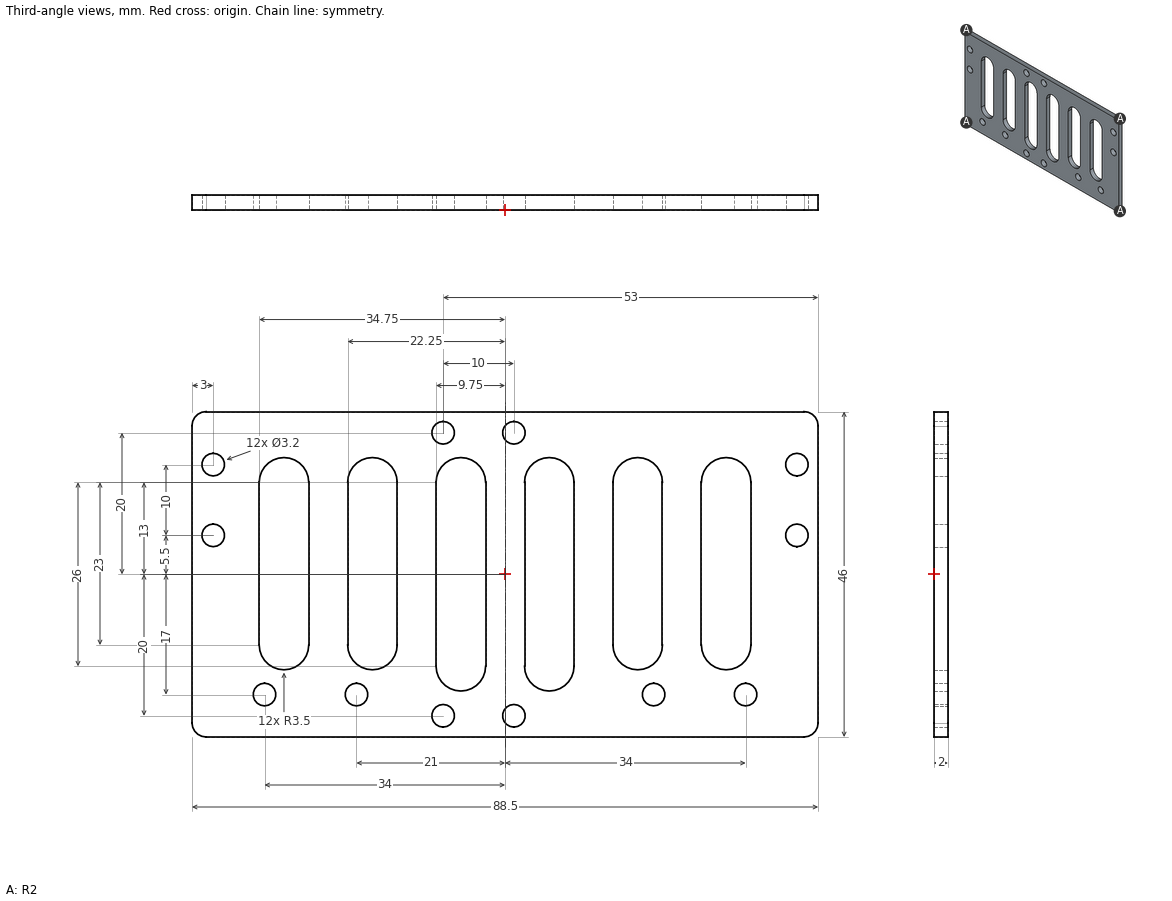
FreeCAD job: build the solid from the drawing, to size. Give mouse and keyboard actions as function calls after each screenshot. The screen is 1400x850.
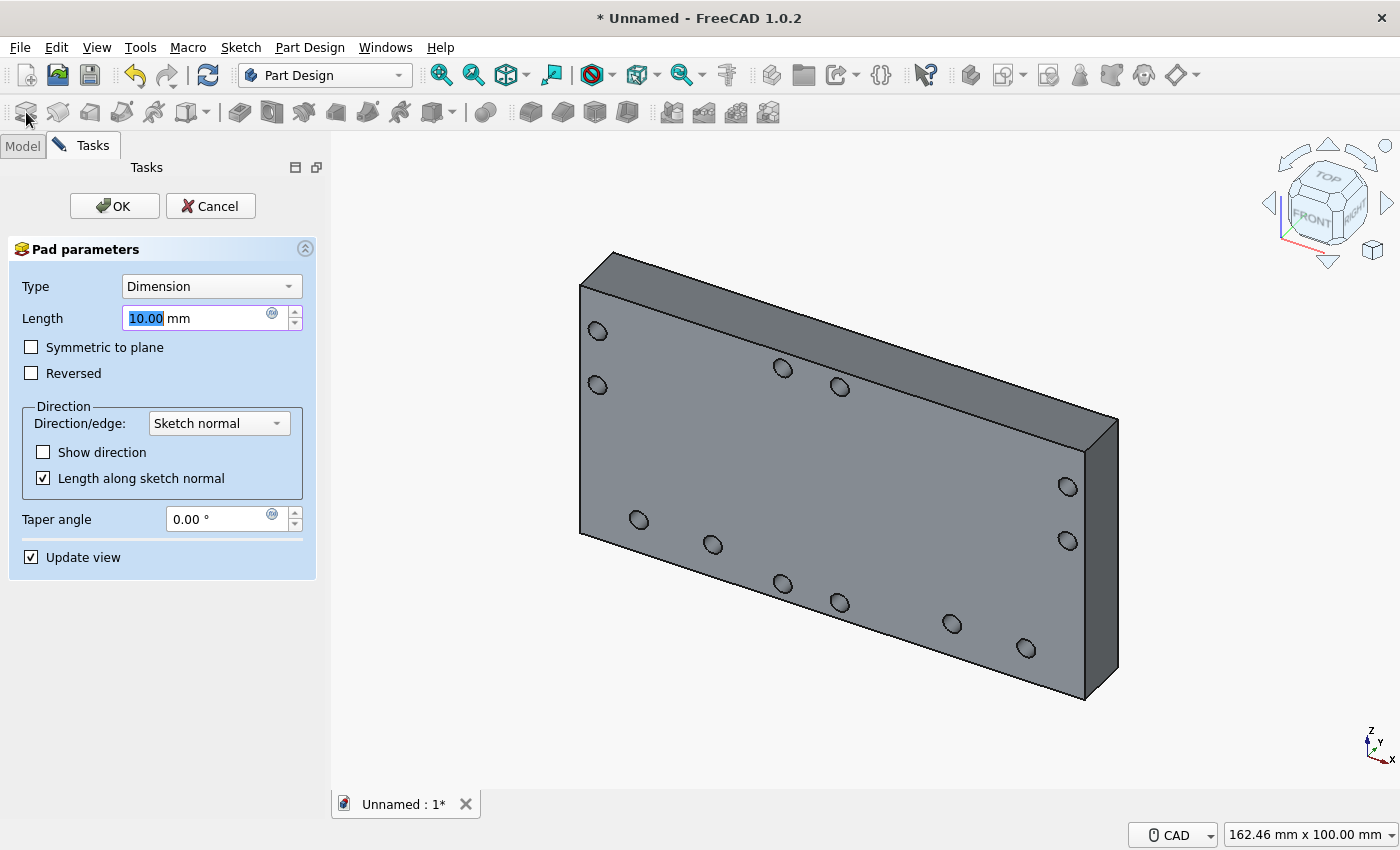
text(2)
key(Tab)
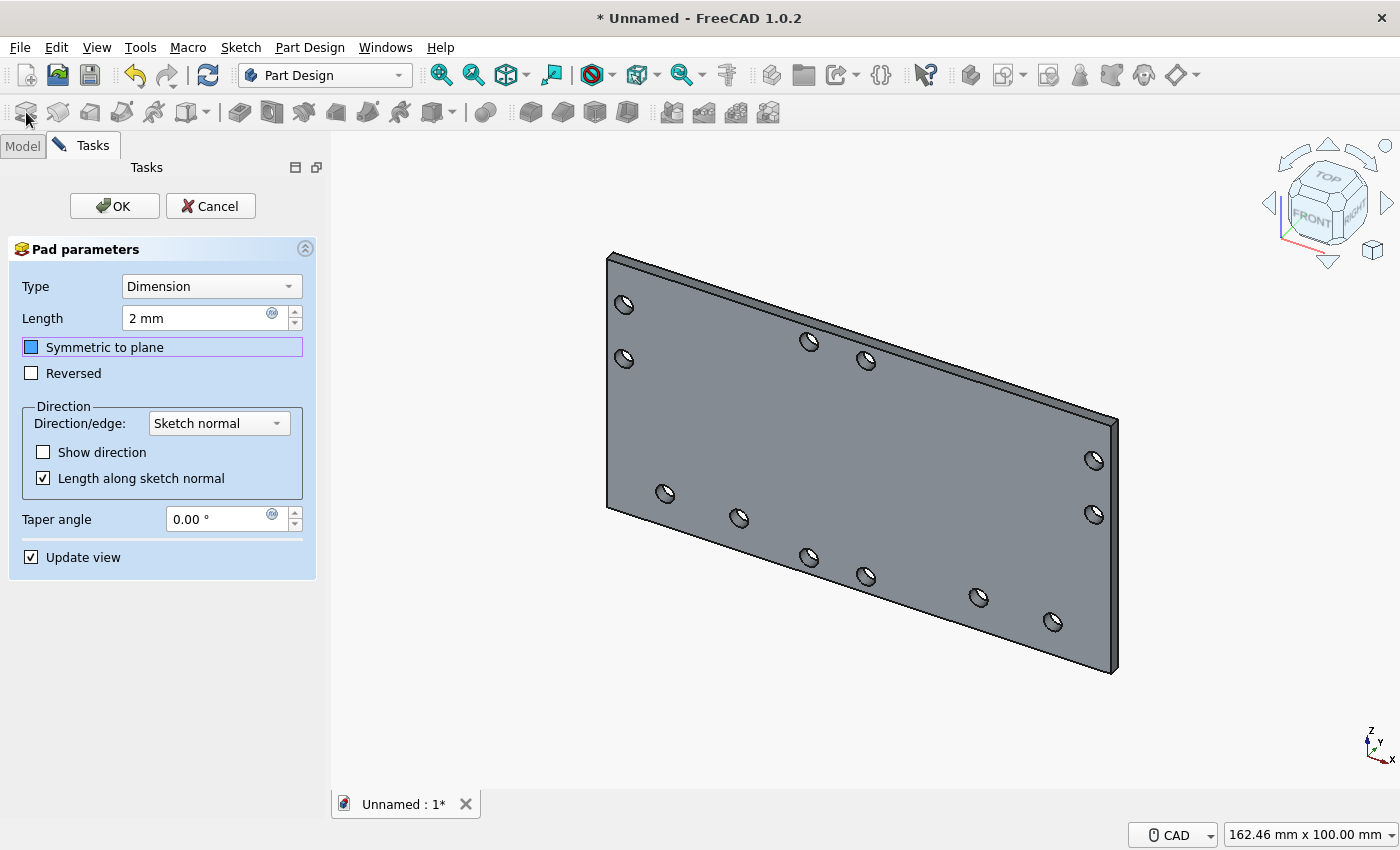
click(30, 373)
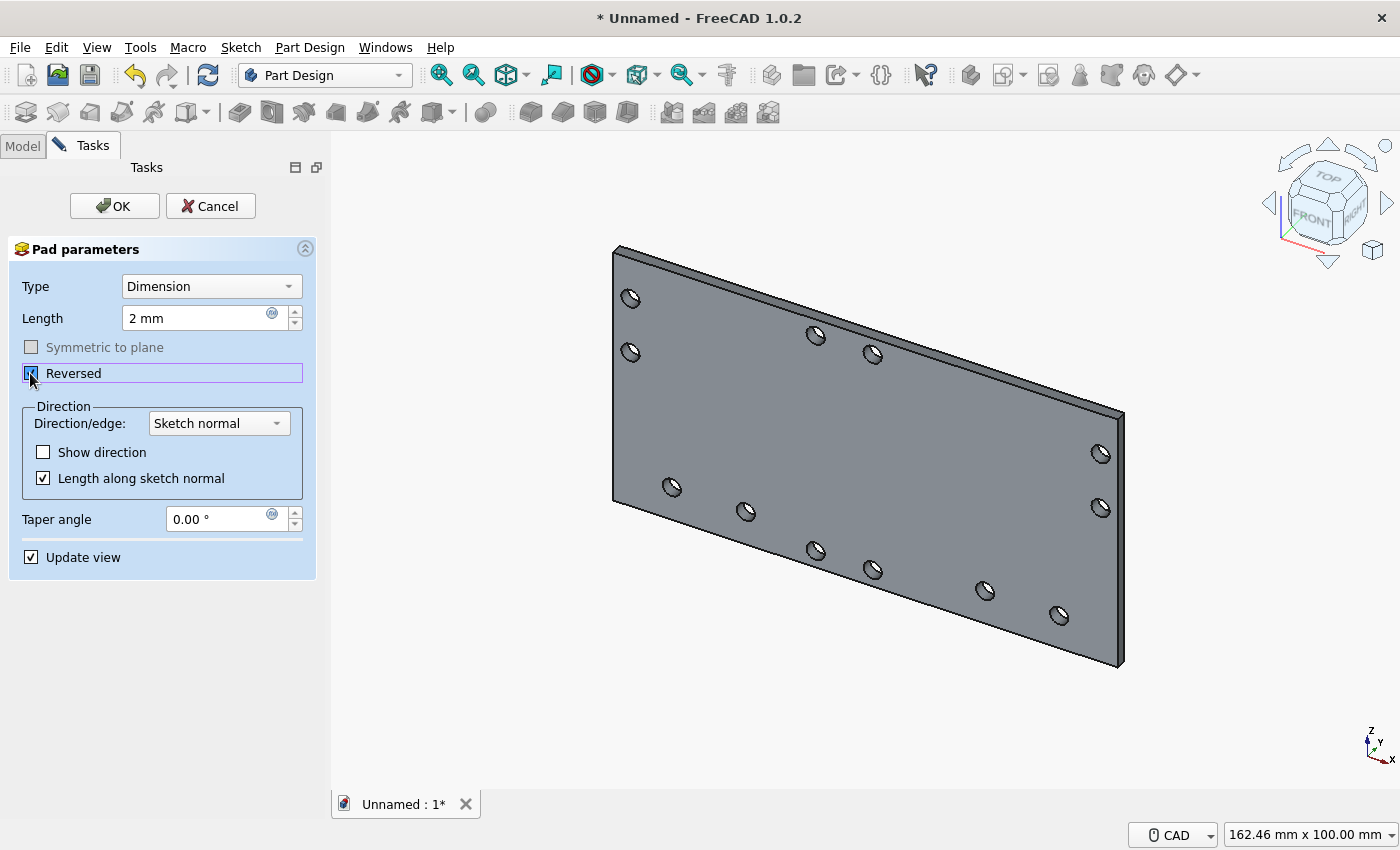
click(115, 206)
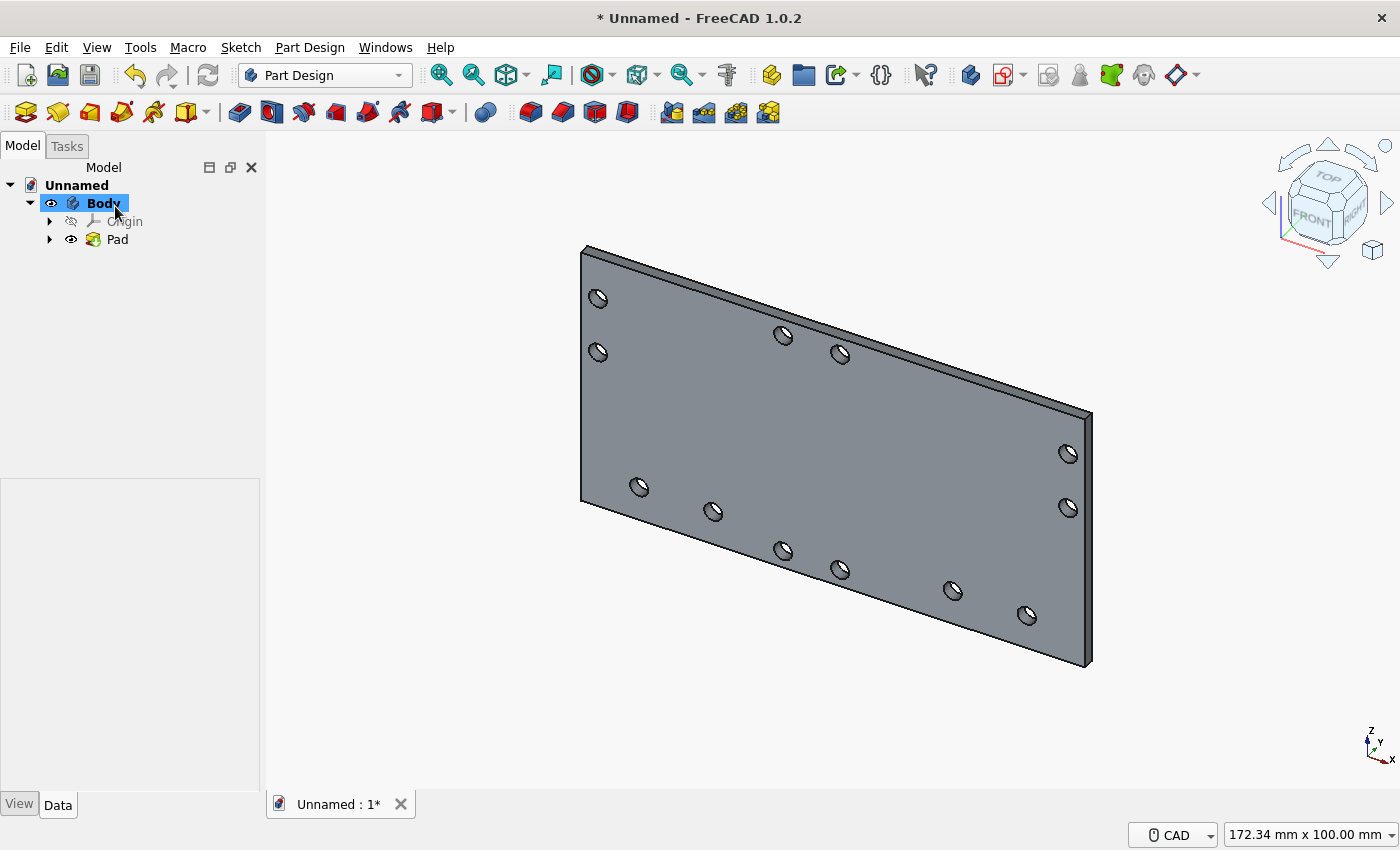
key(4)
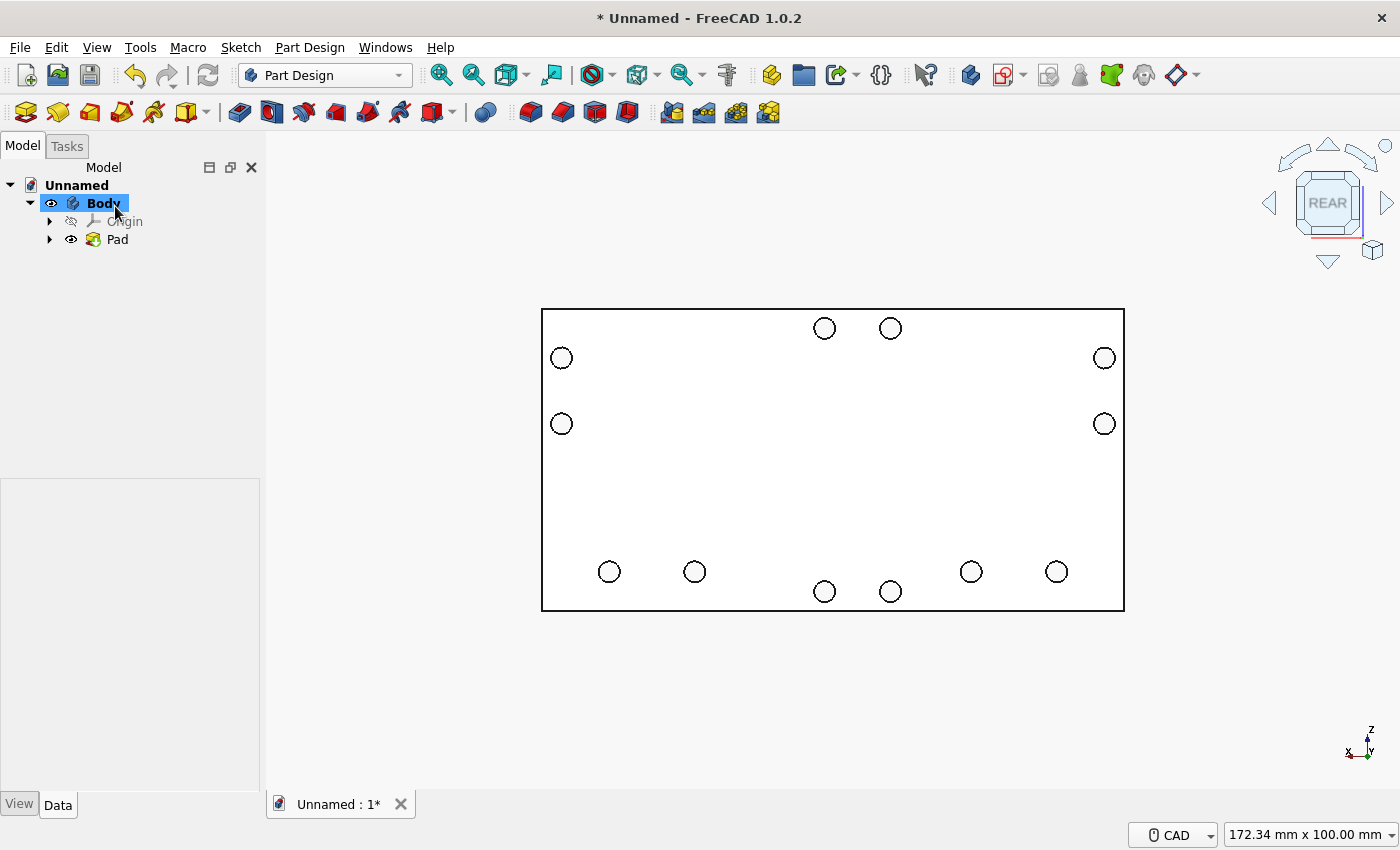
click(833, 459)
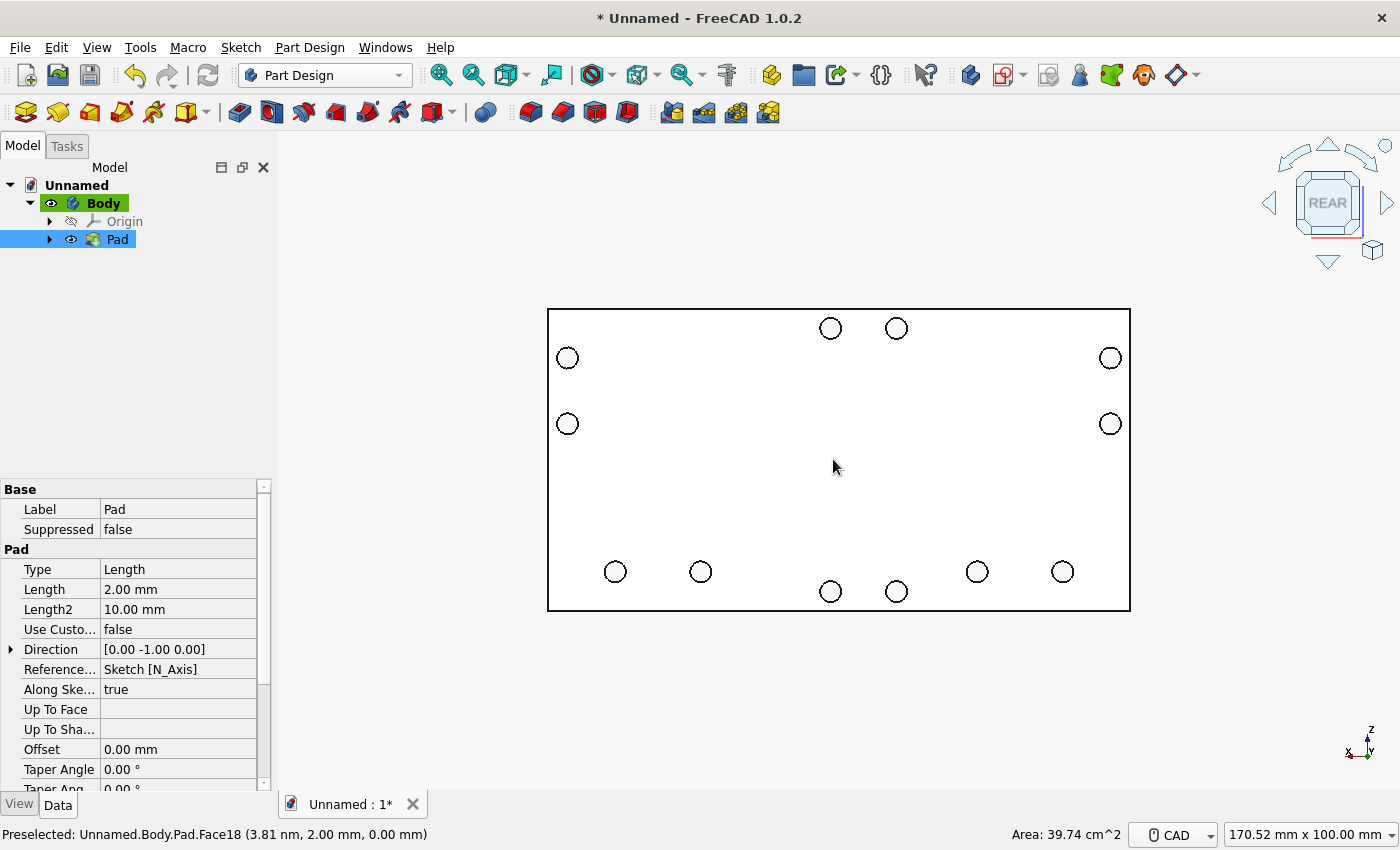
click(1004, 76)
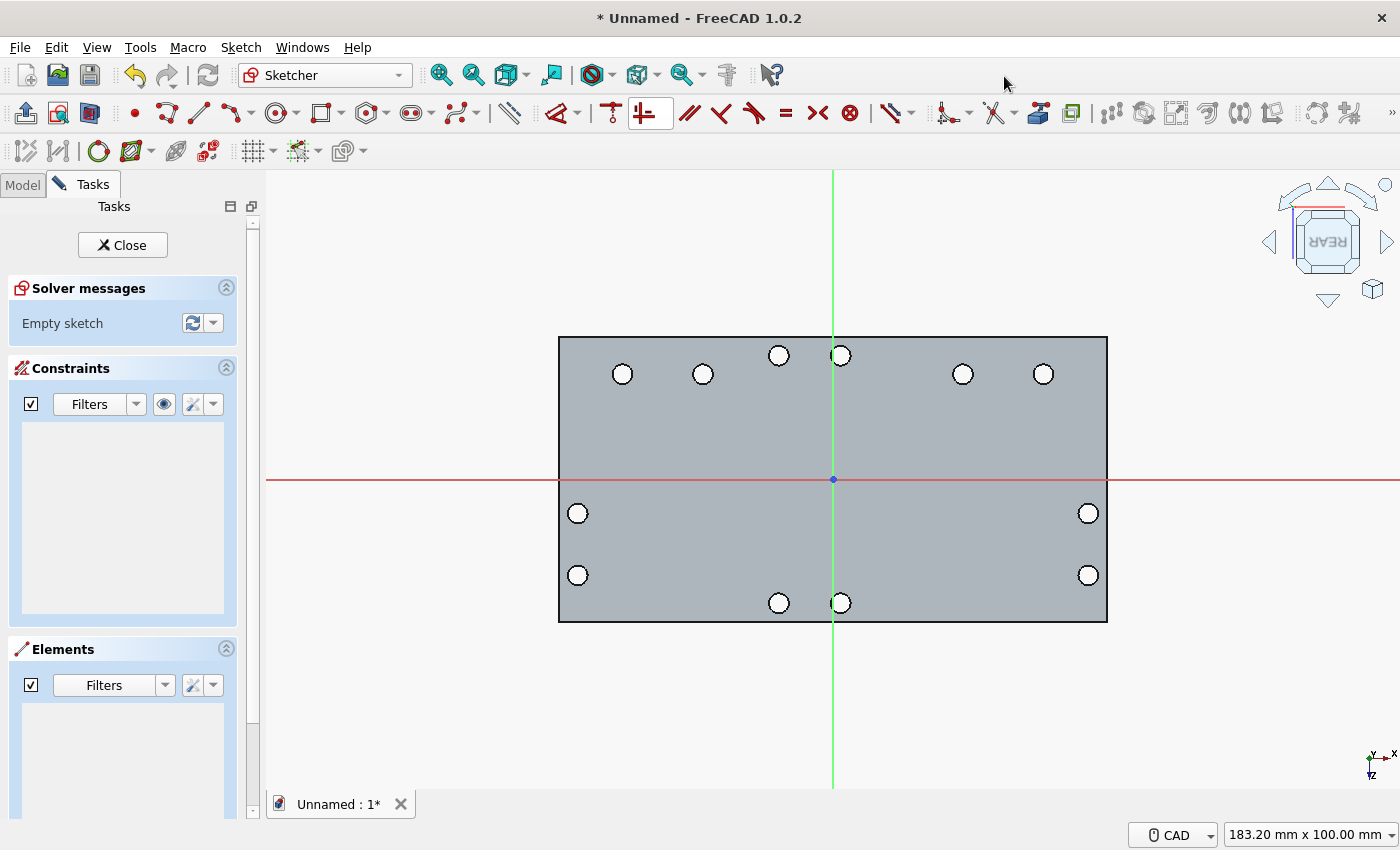
scroll(972, 480, up, 2)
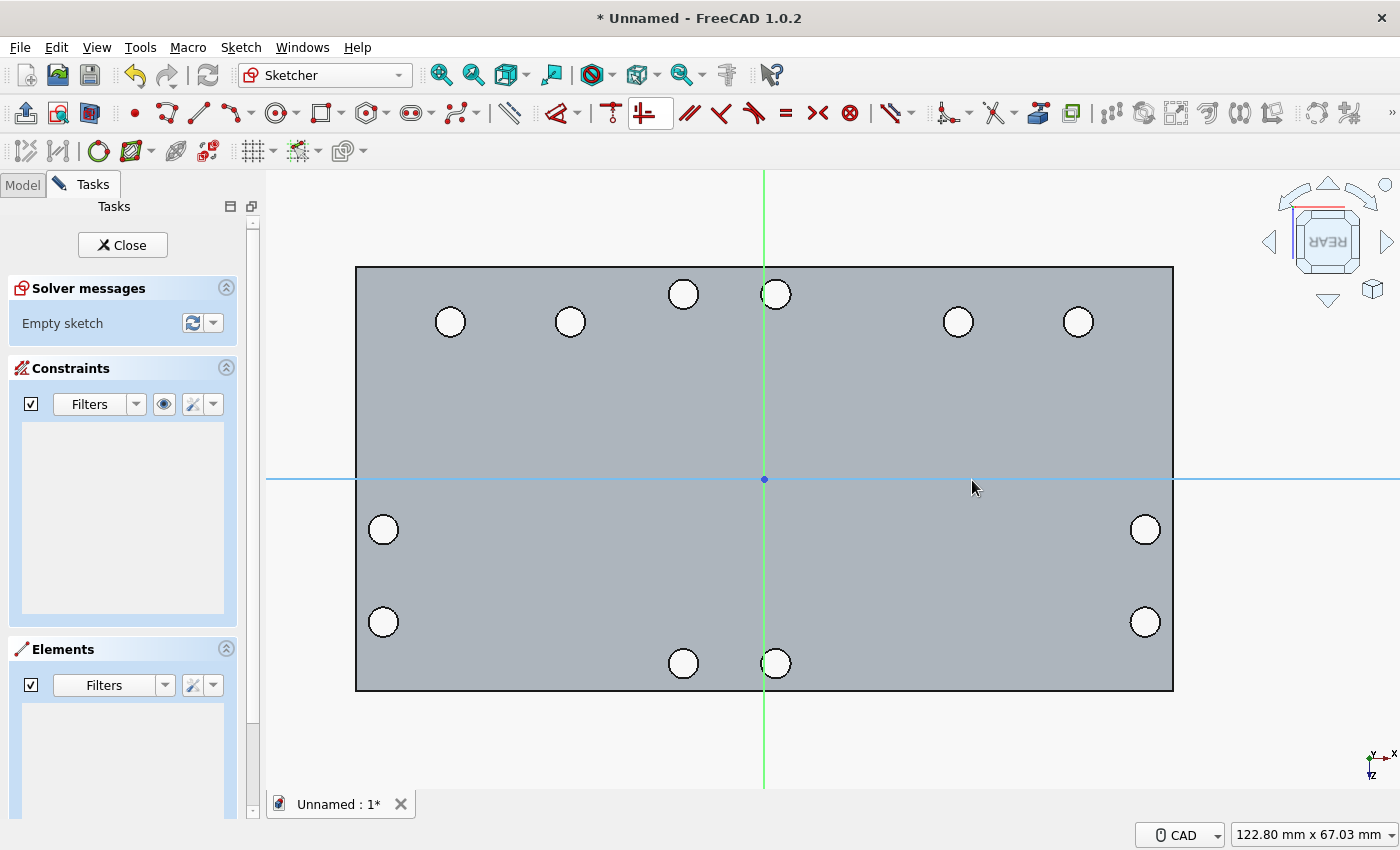
click(412, 114)